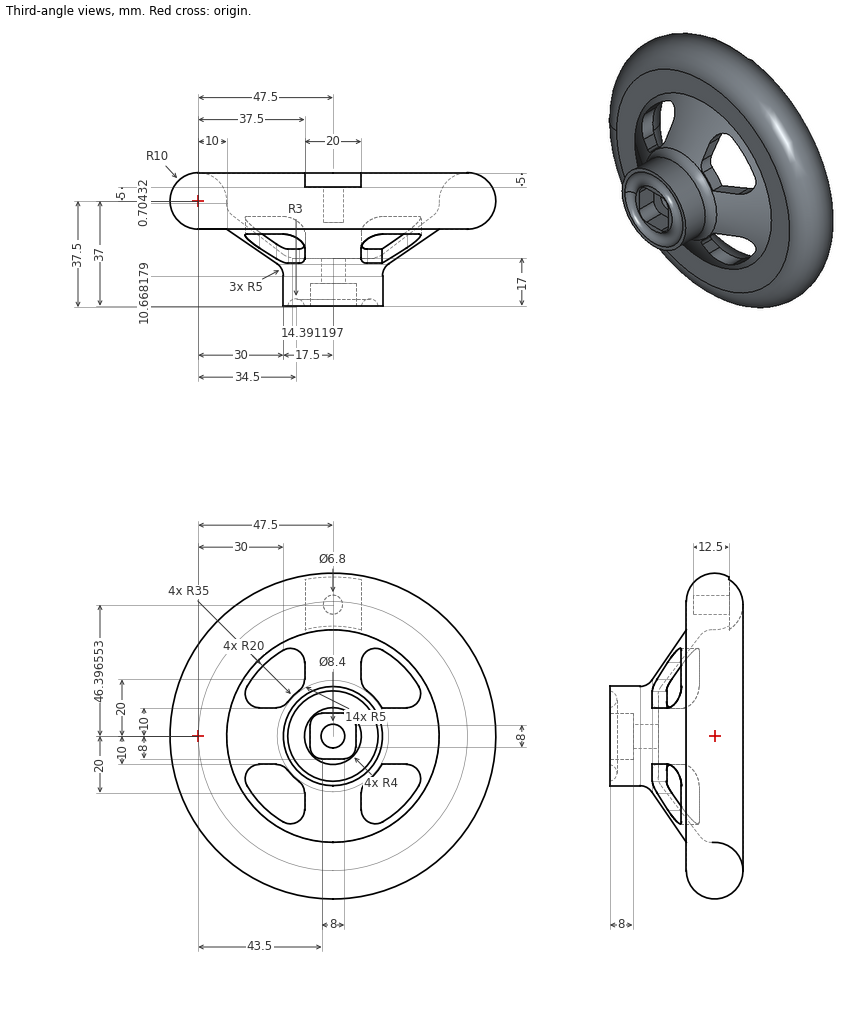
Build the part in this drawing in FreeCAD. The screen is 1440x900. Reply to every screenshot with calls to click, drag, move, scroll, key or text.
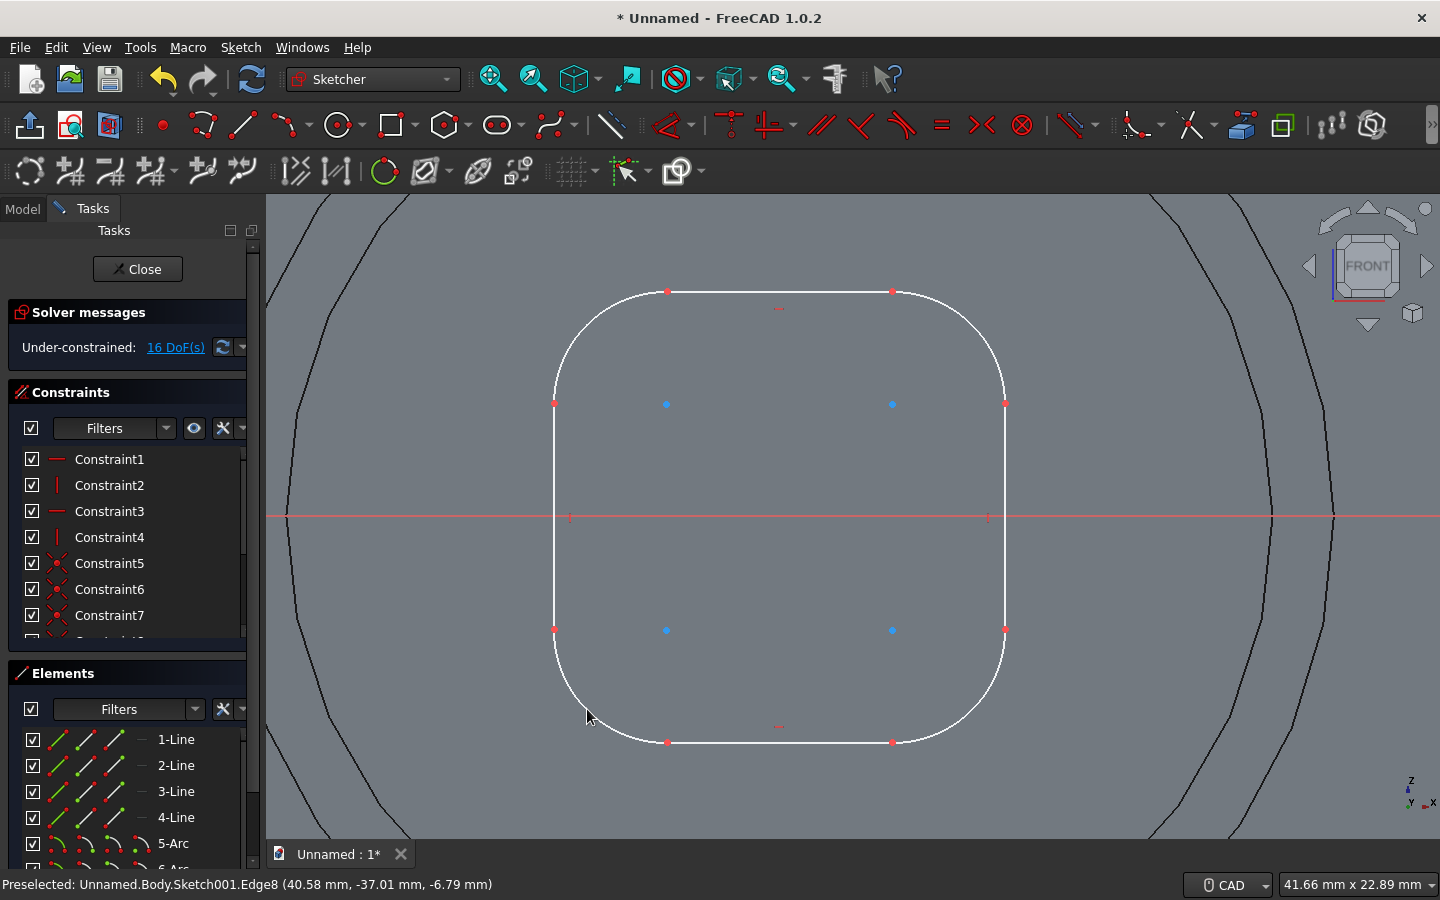
click(734, 743)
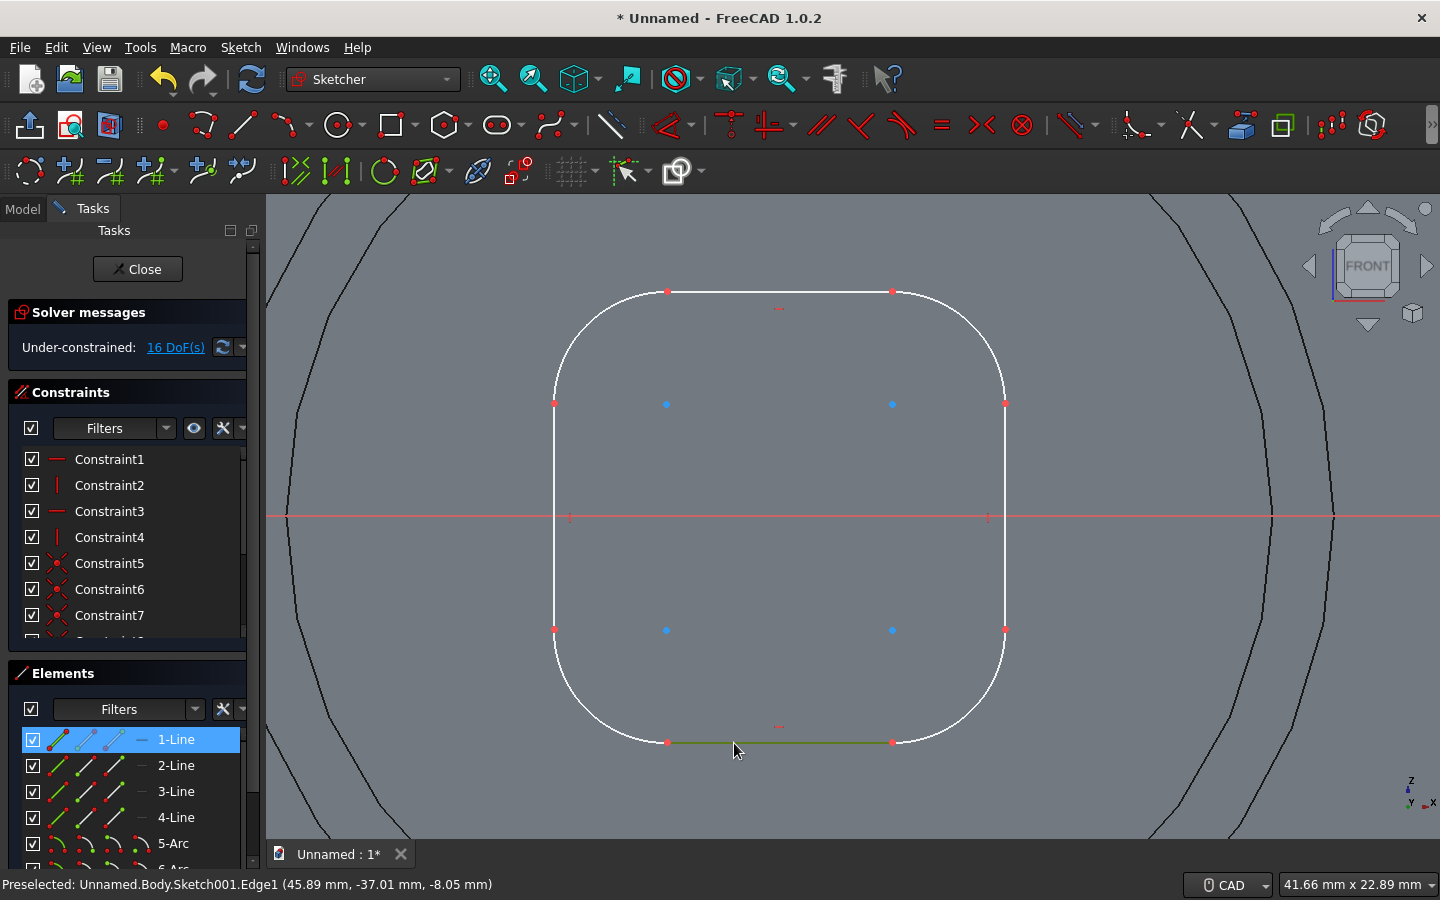
click(943, 731)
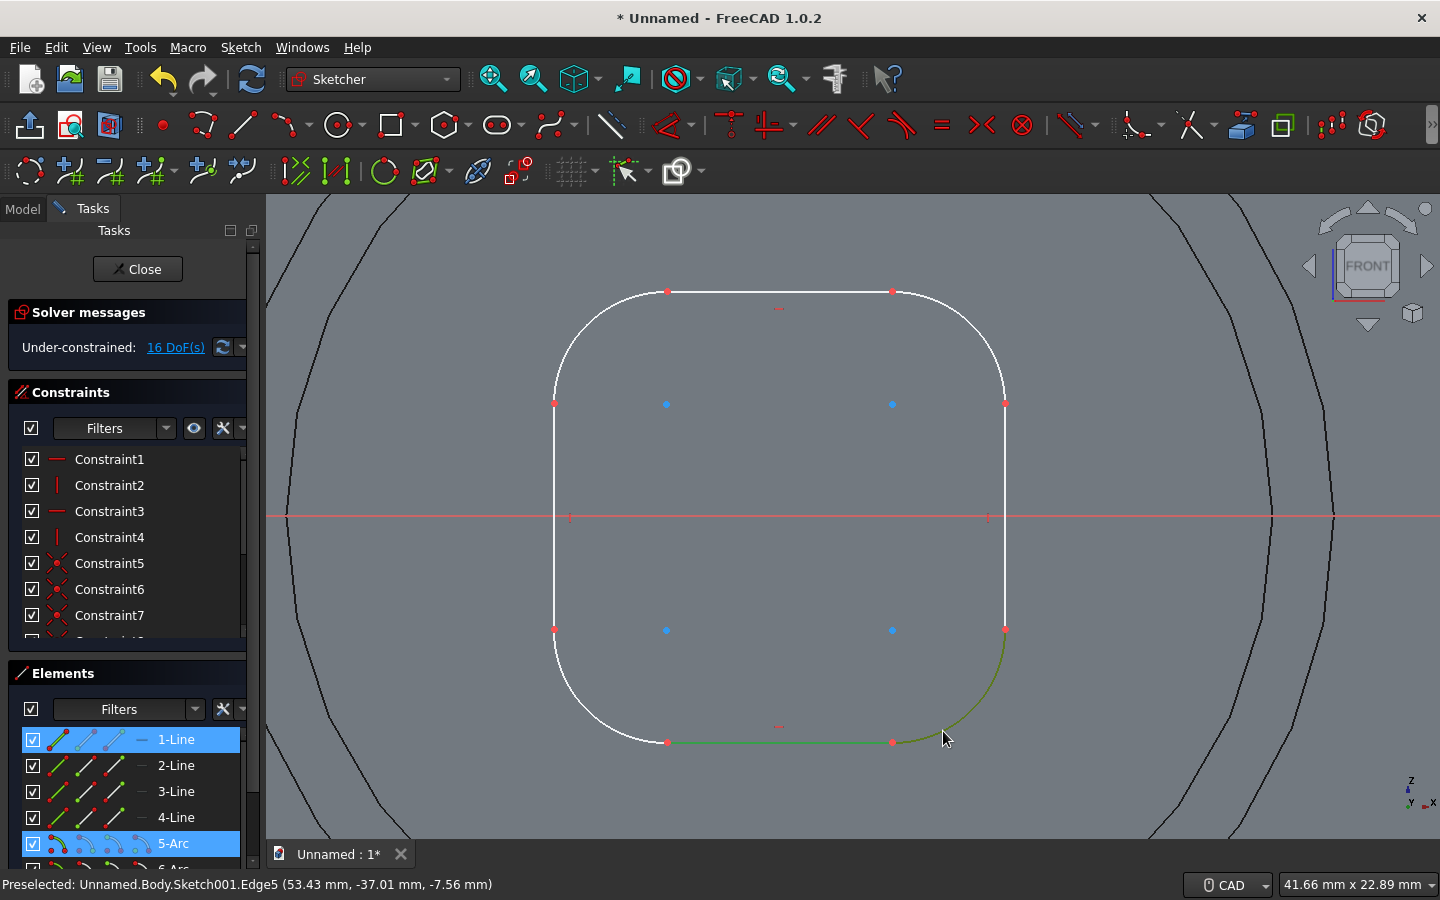
click(902, 126)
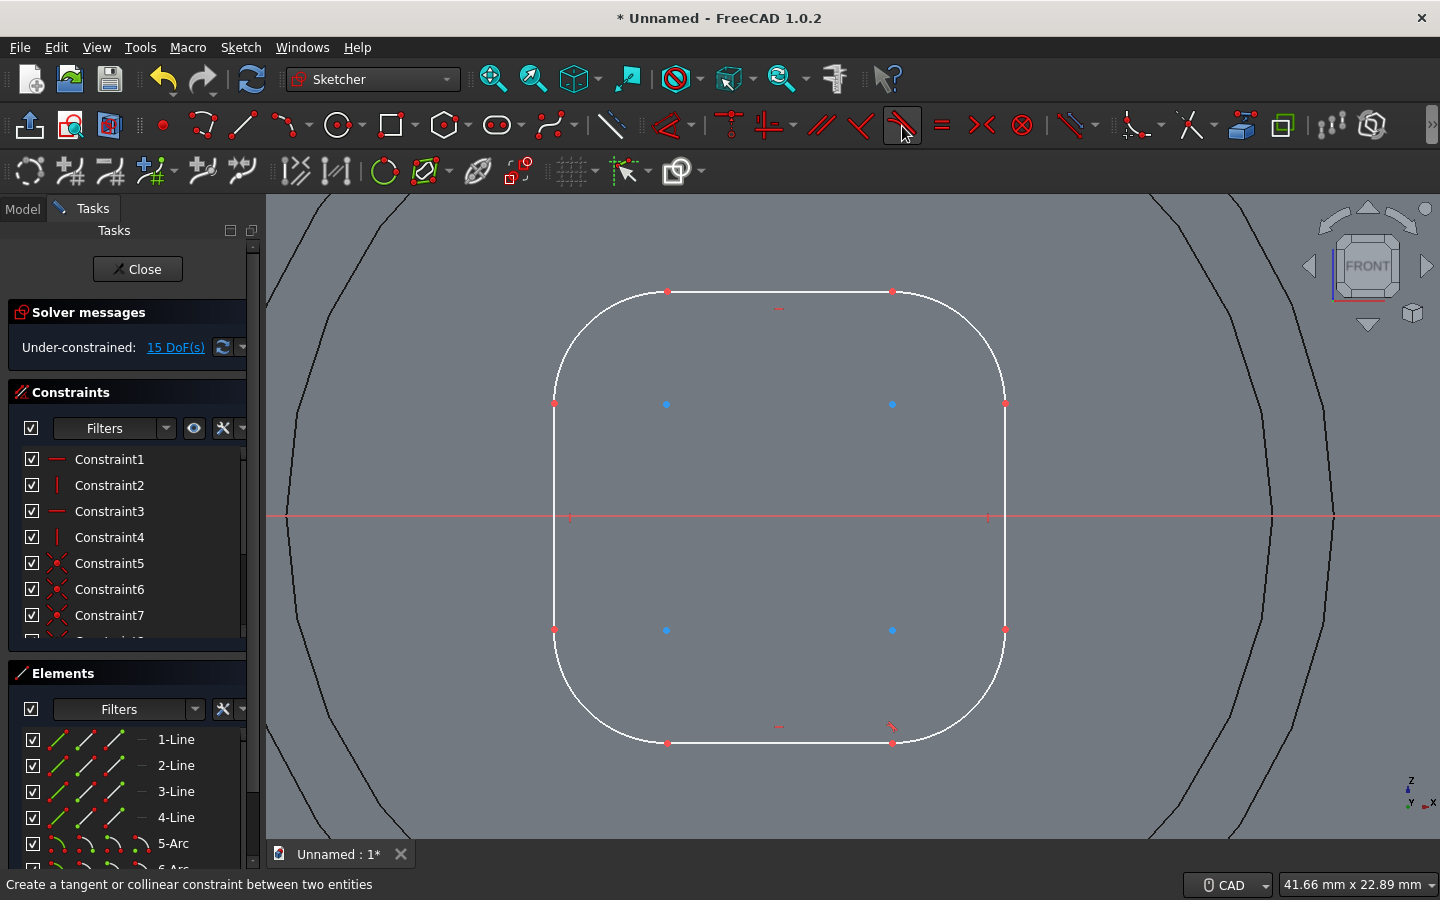
click(734, 743)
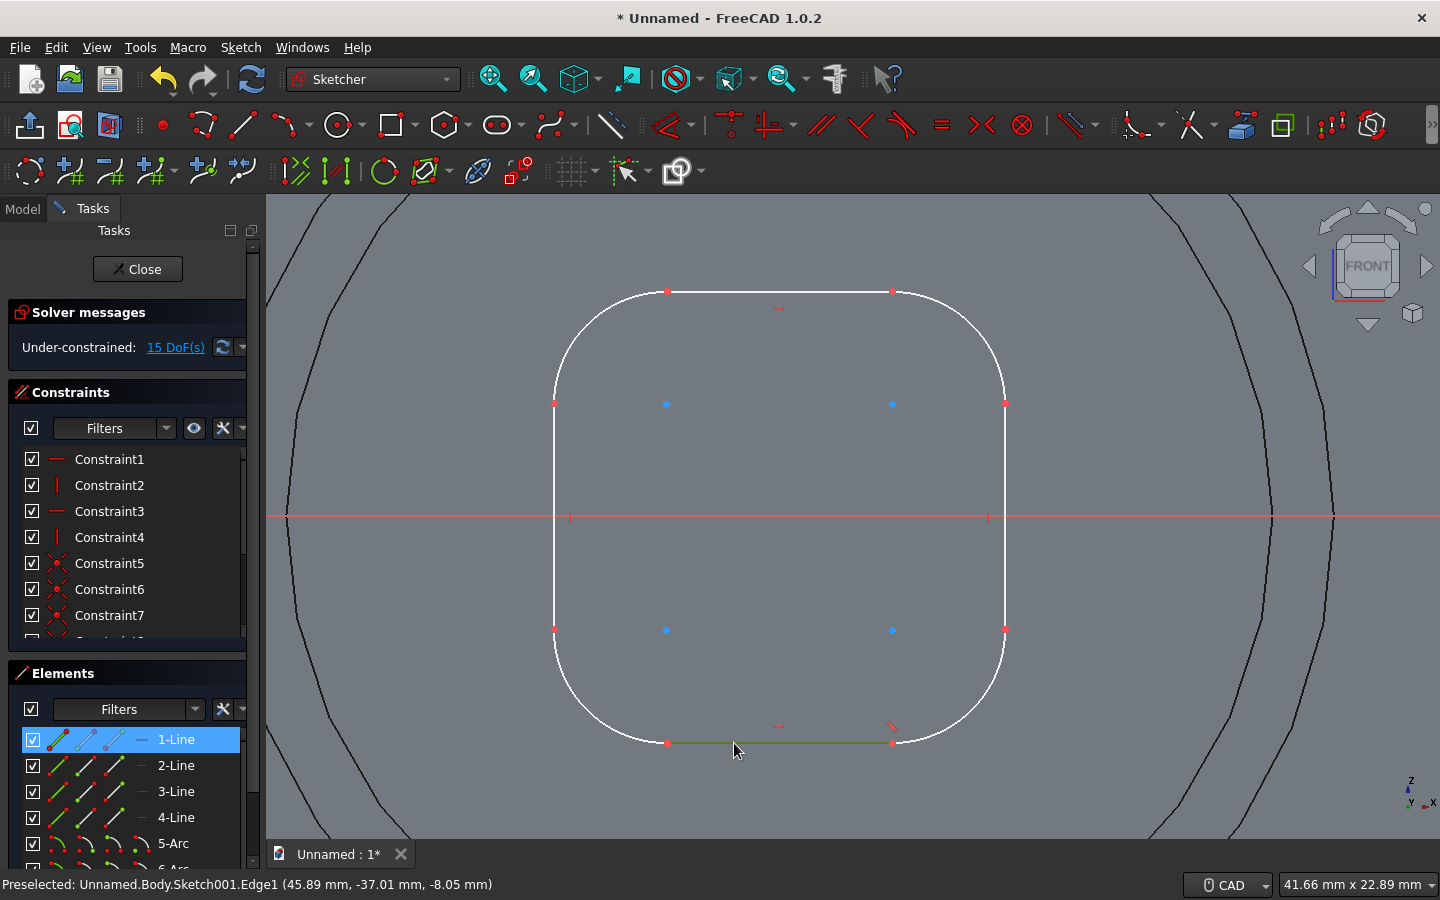
click(566, 681)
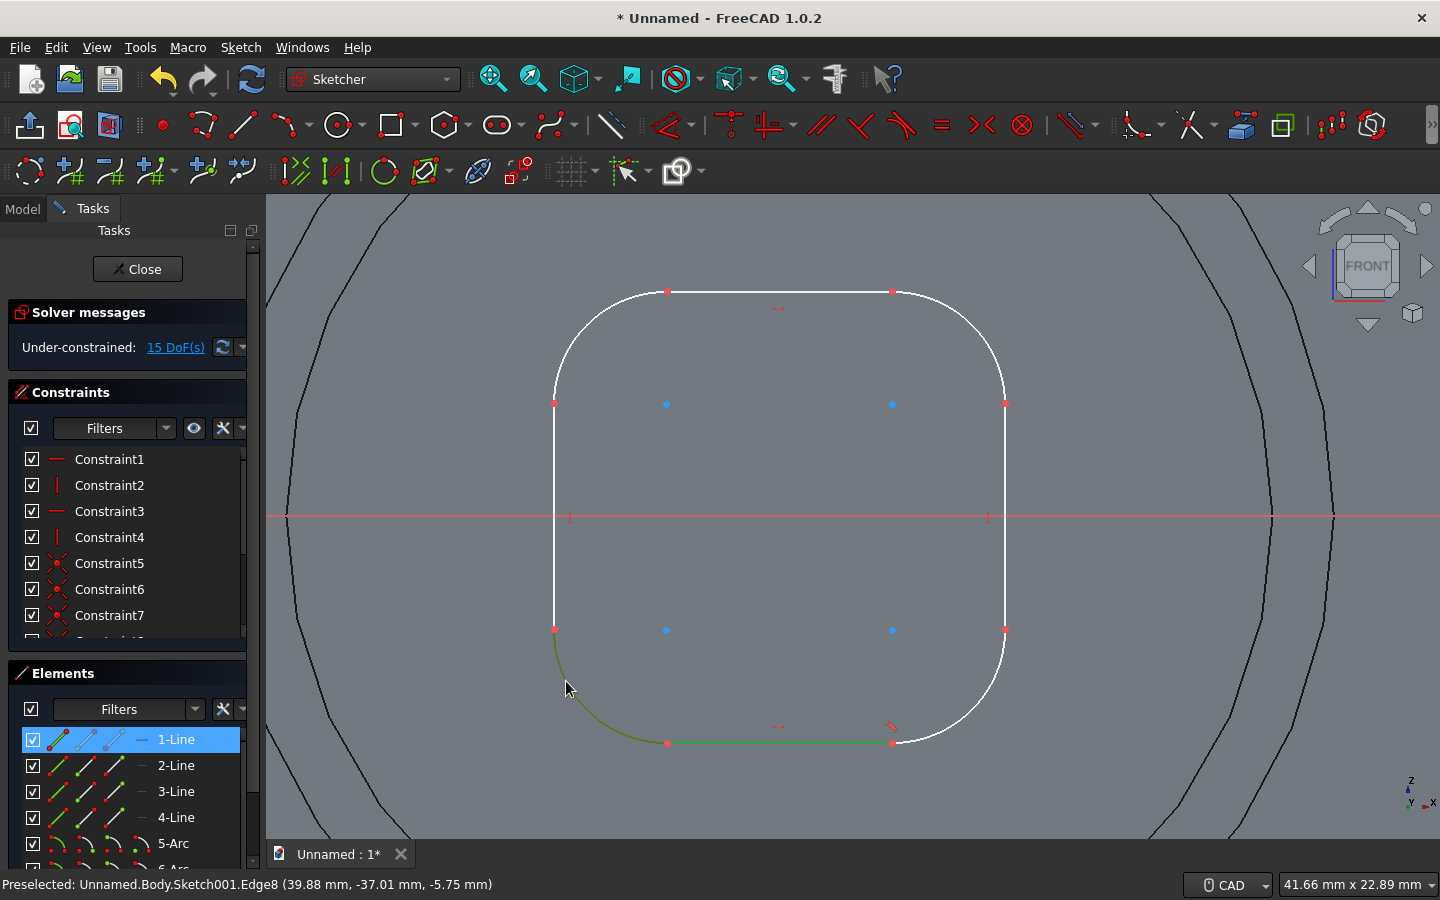
click(902, 126)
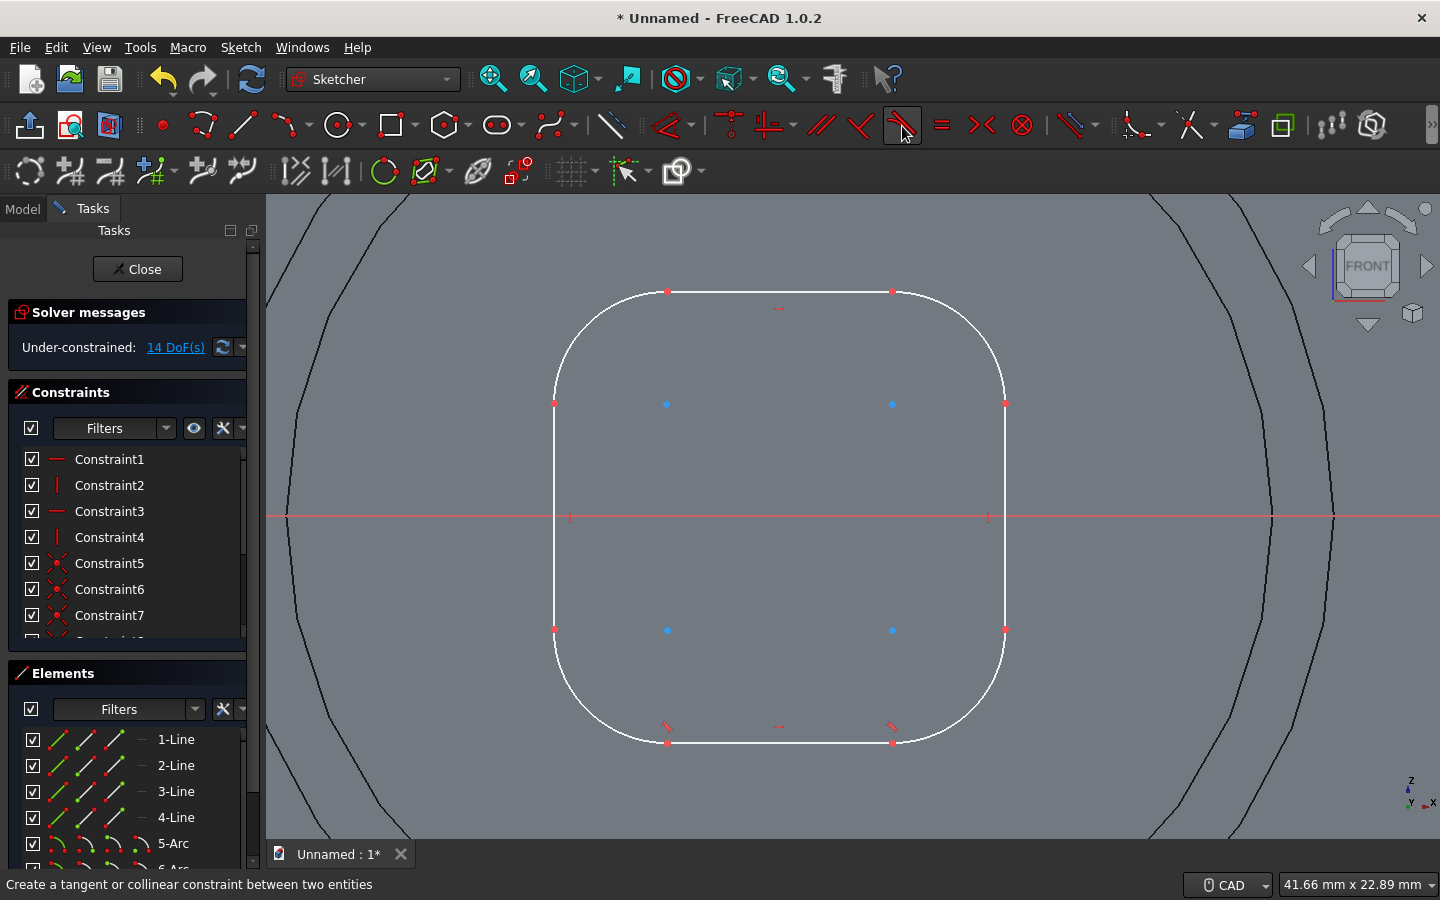
click(1005, 562)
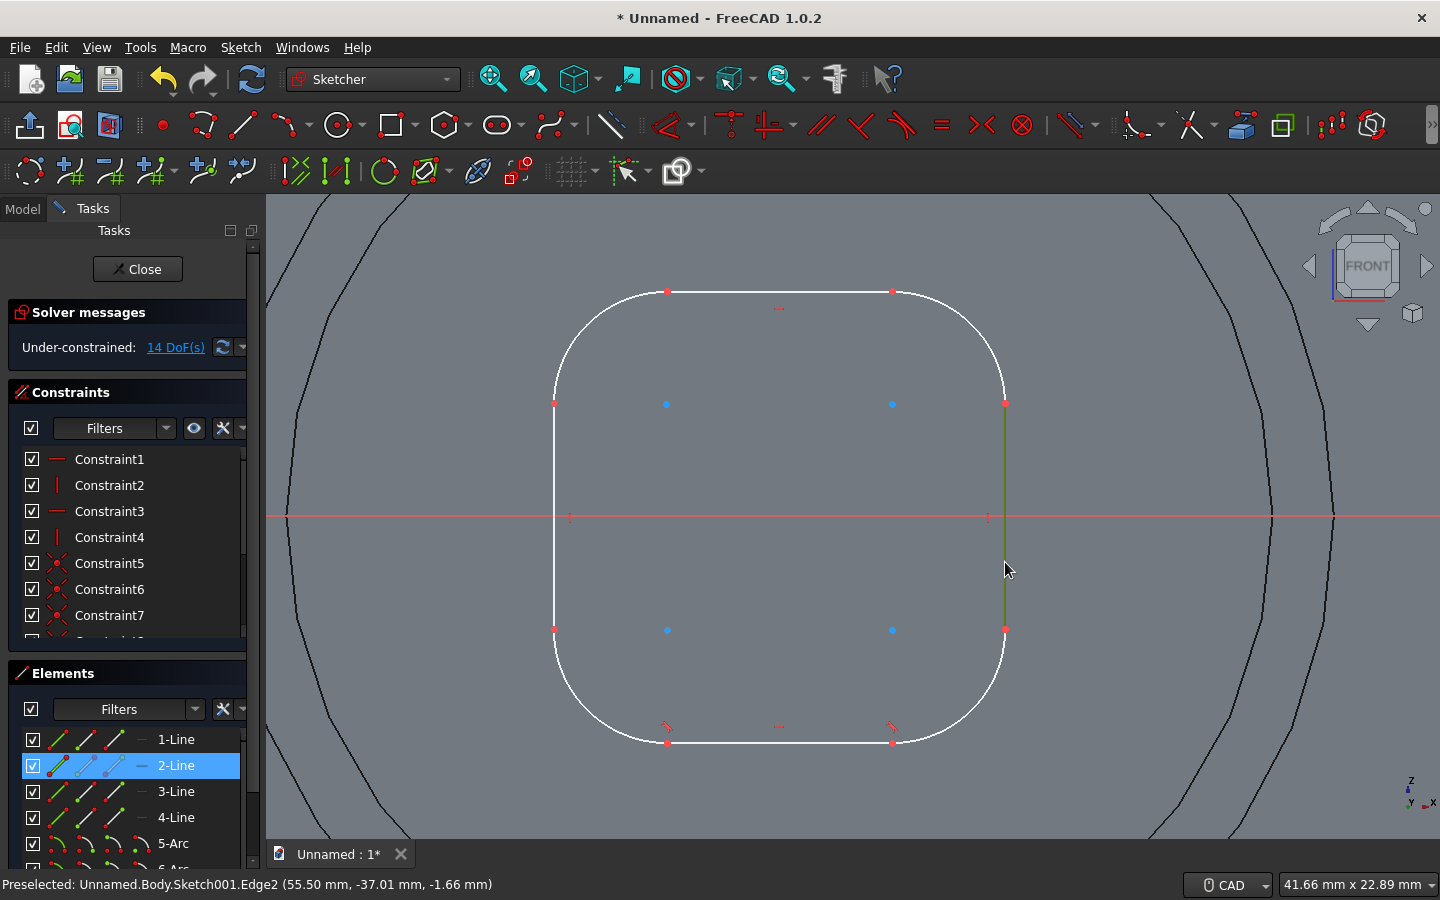
click(943, 731)